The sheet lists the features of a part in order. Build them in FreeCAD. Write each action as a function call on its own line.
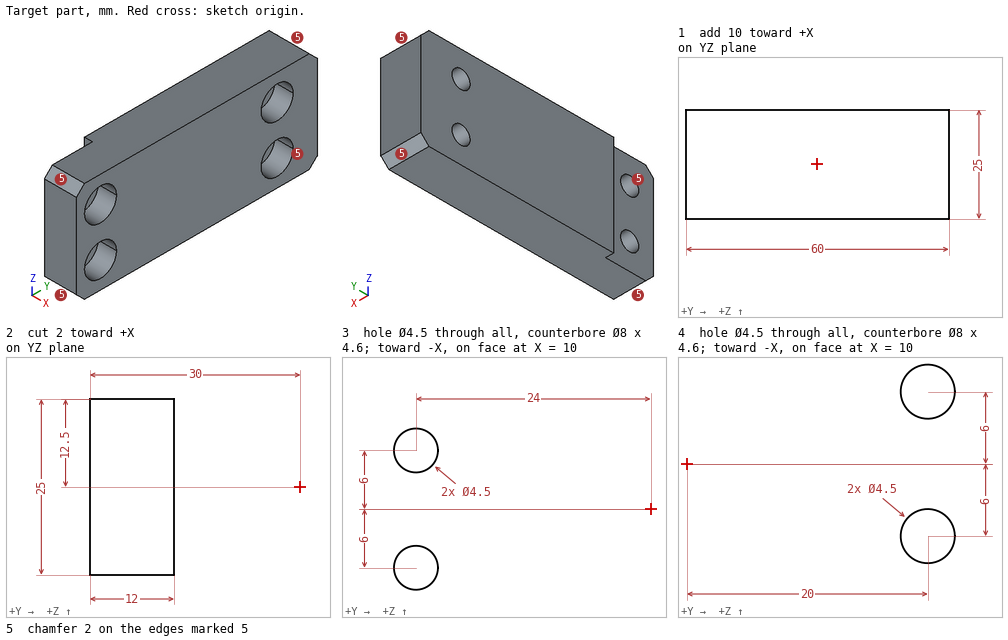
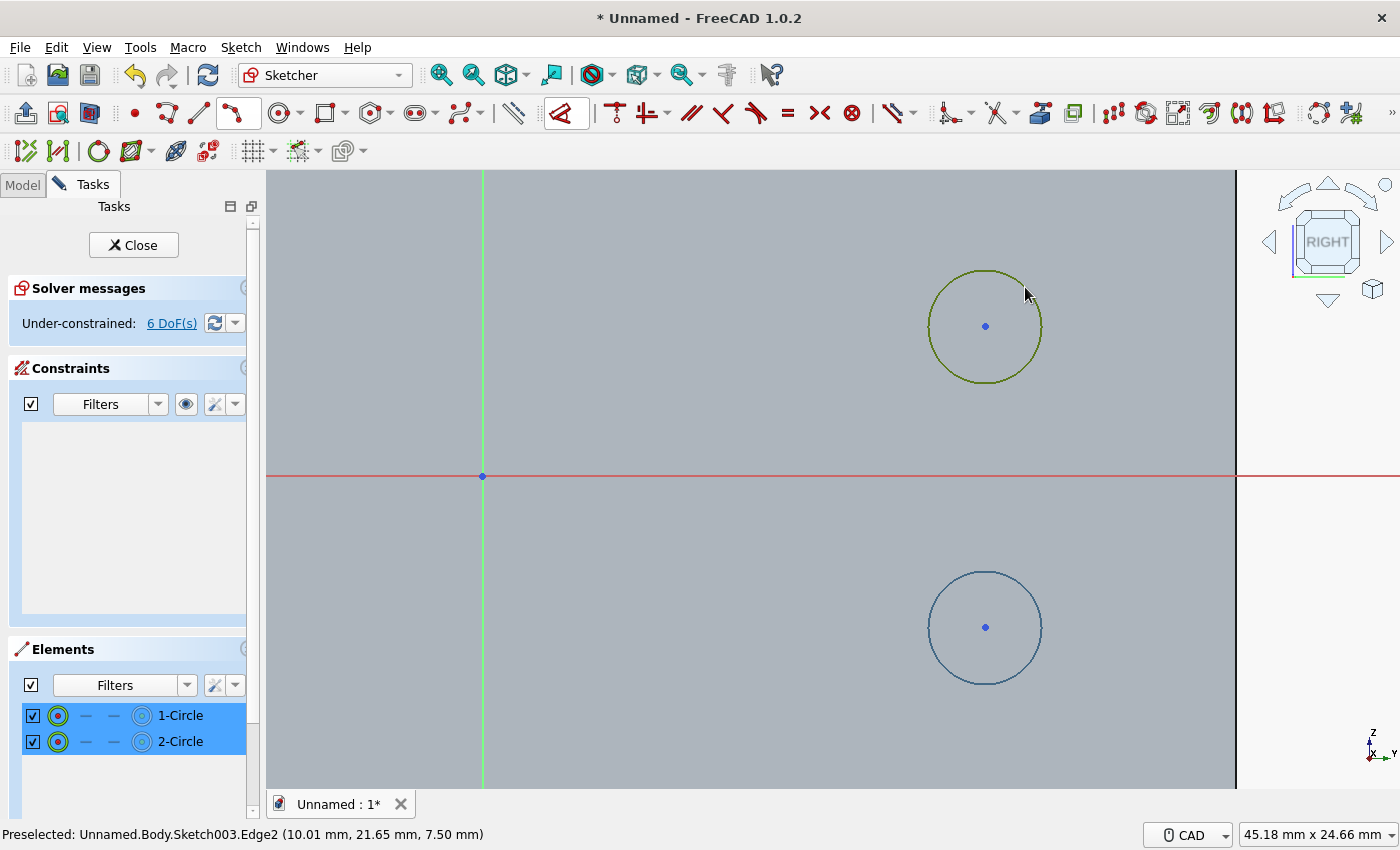
key(e)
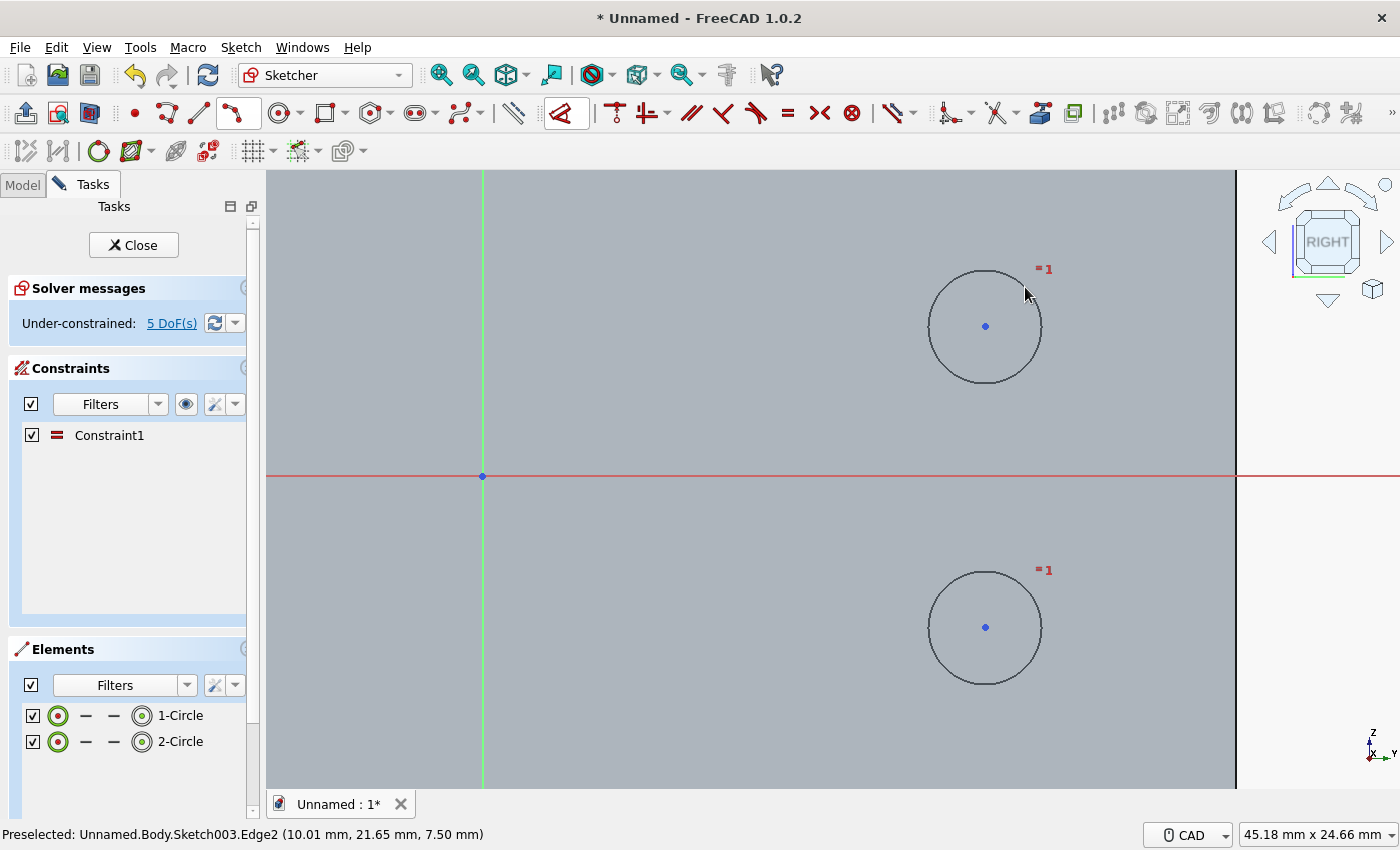
click(985, 628)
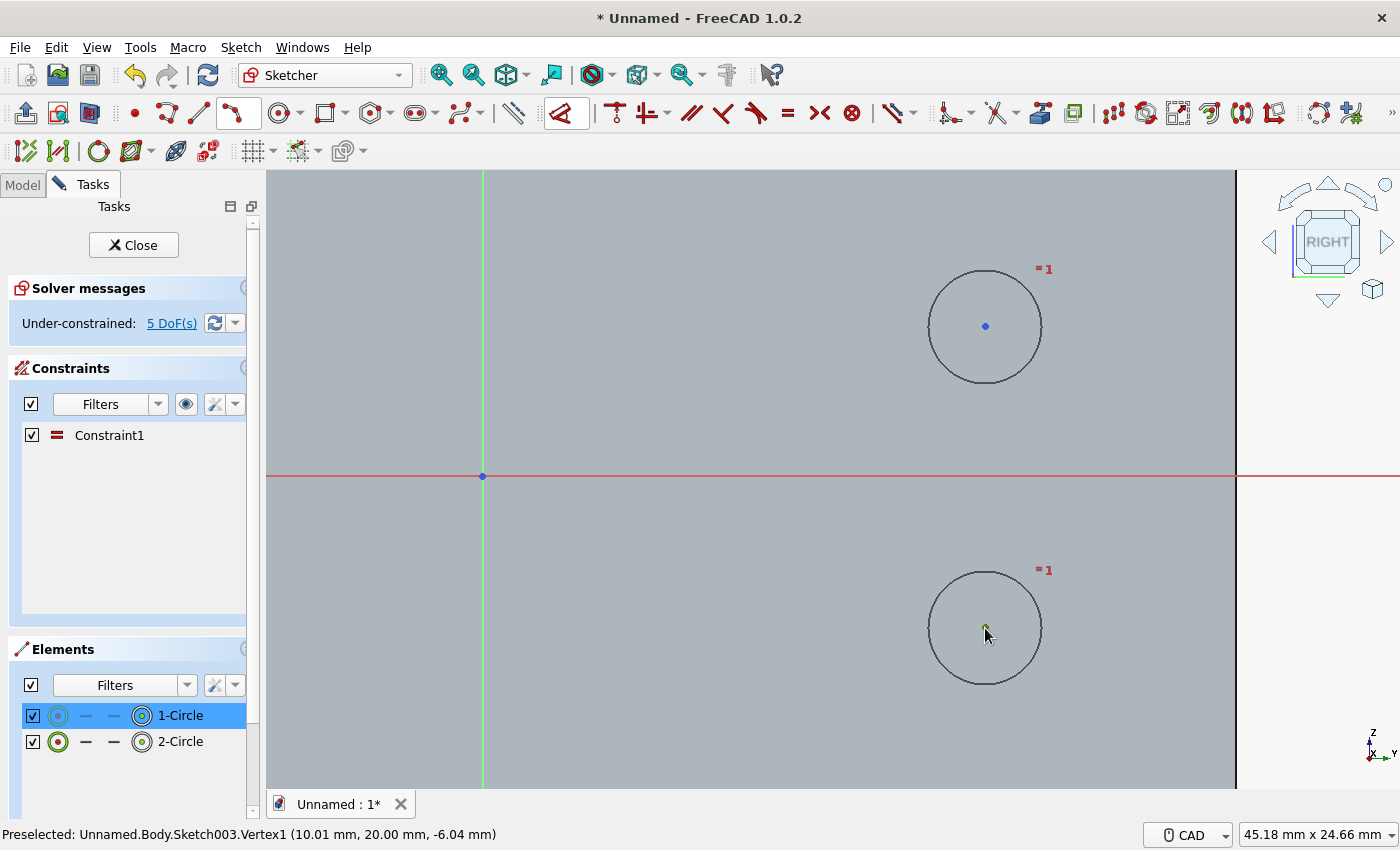
click(985, 327)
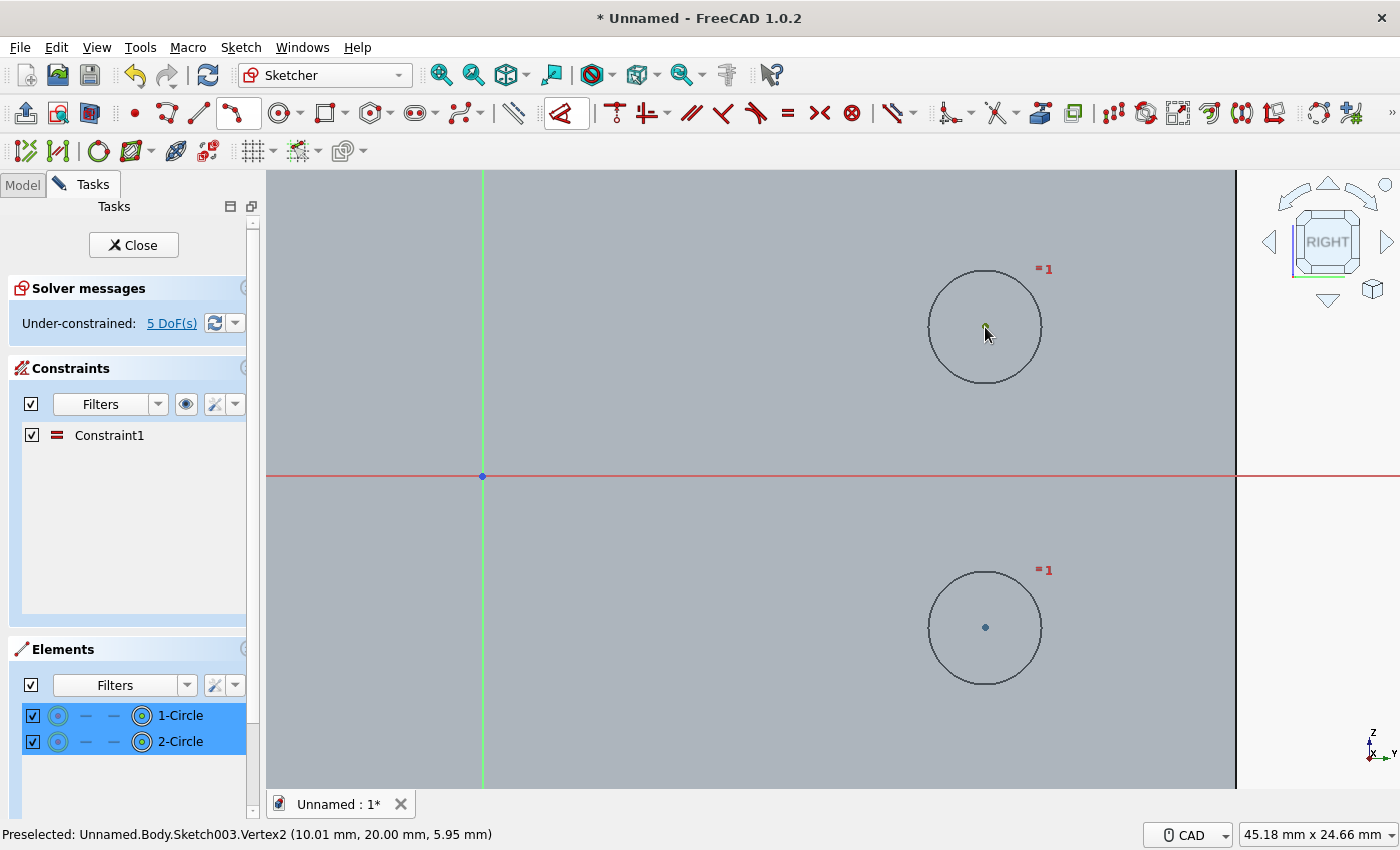
click(670, 114)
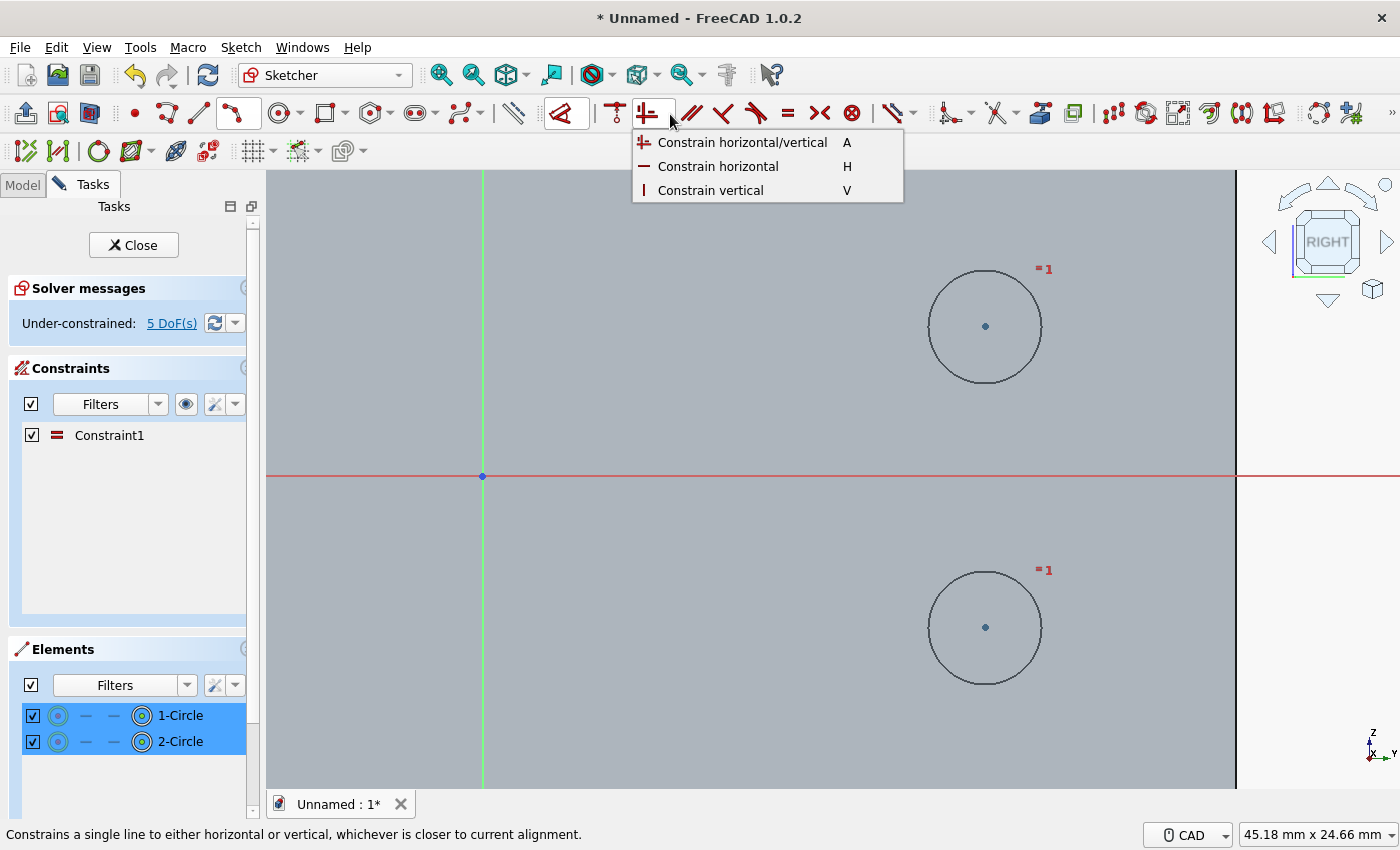
click(768, 190)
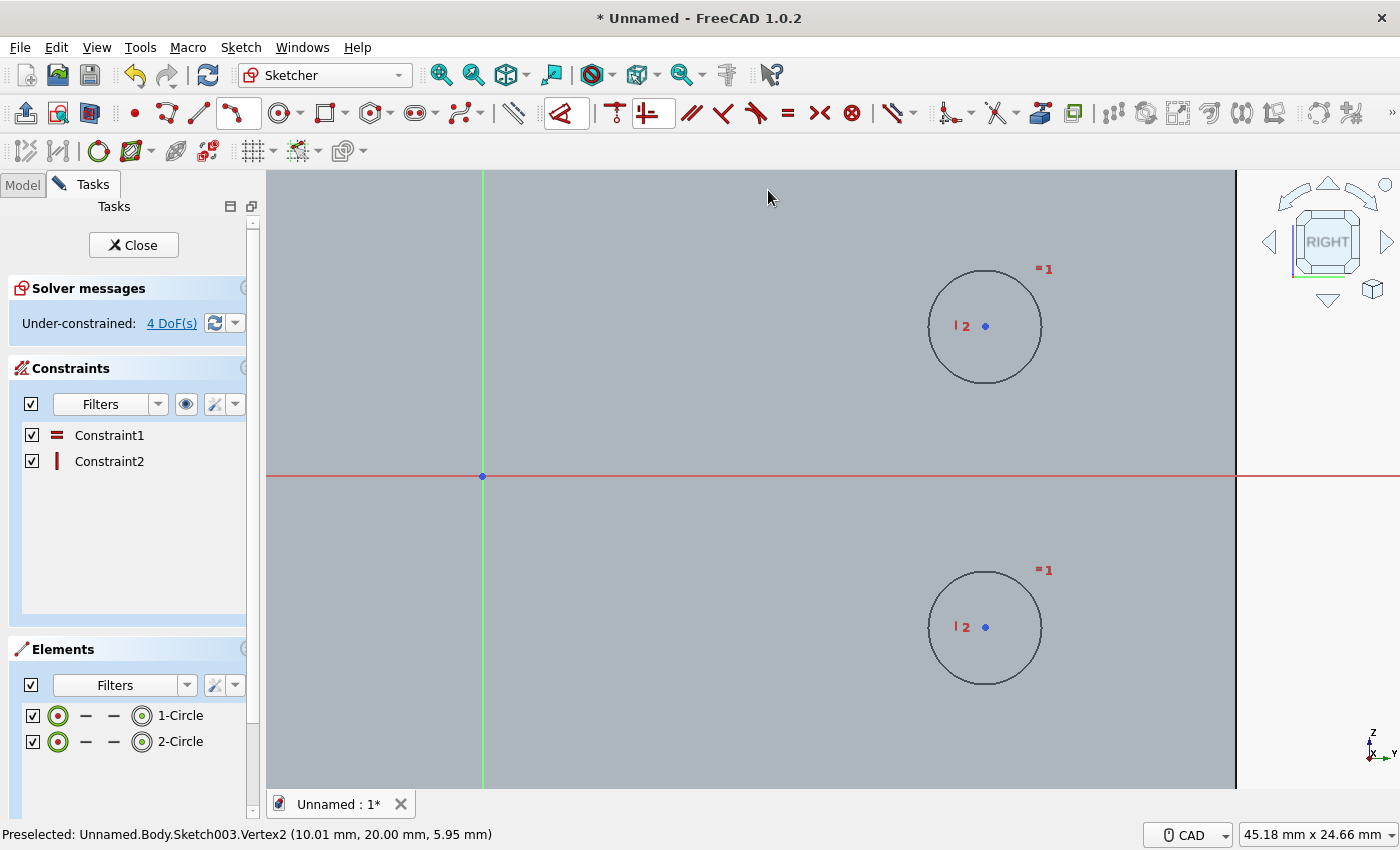
click(1025, 588)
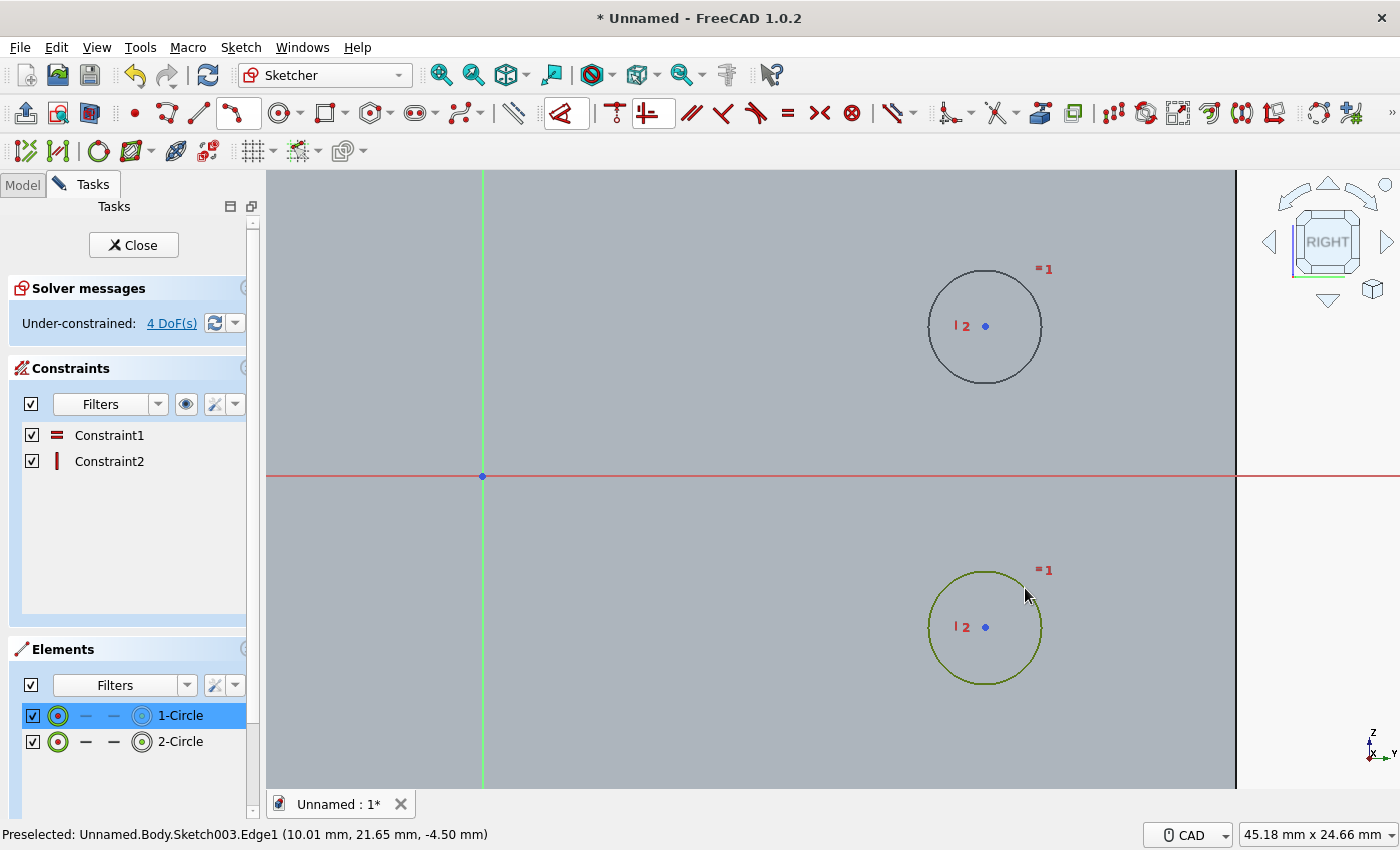
click(584, 114)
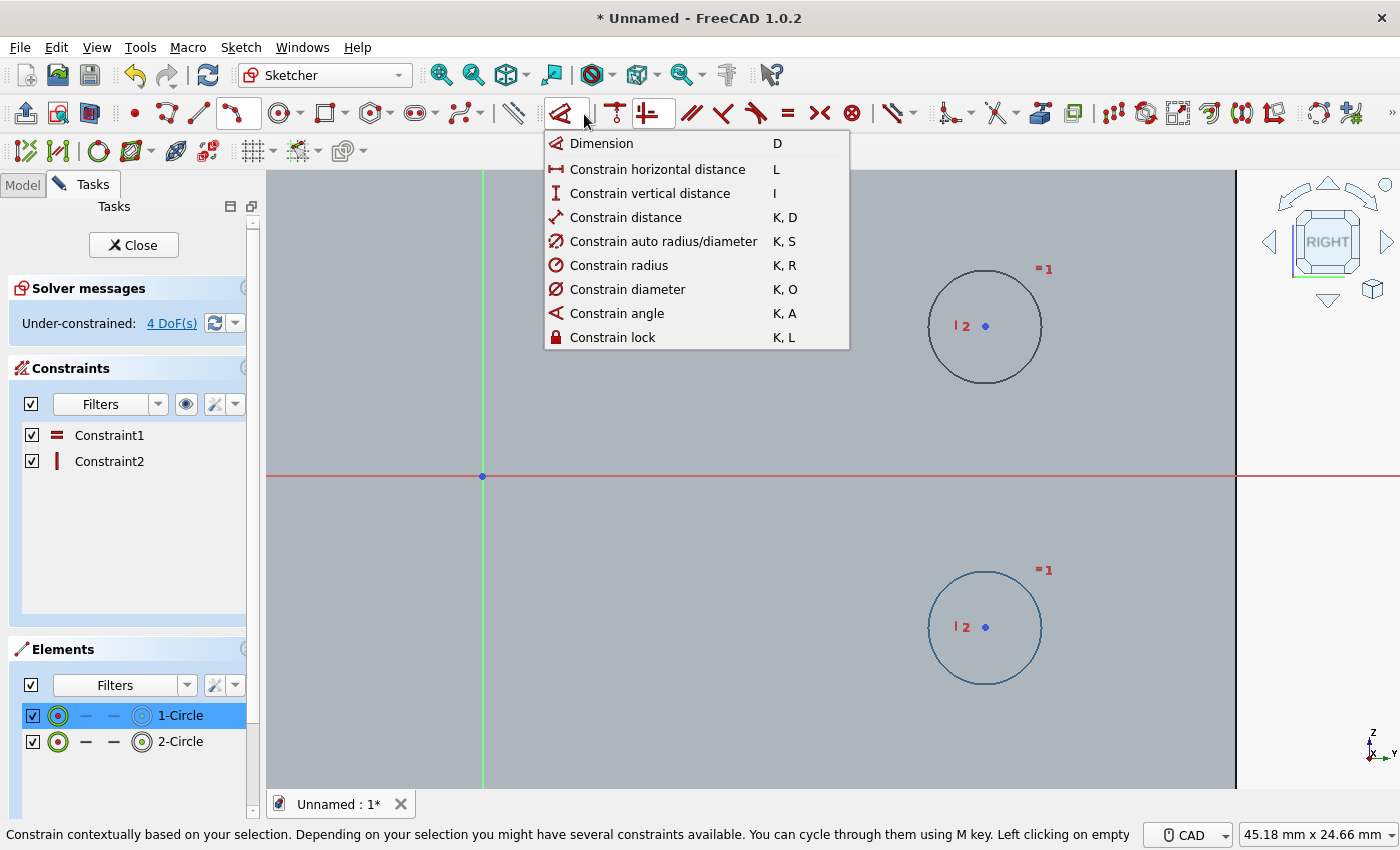
click(697, 289)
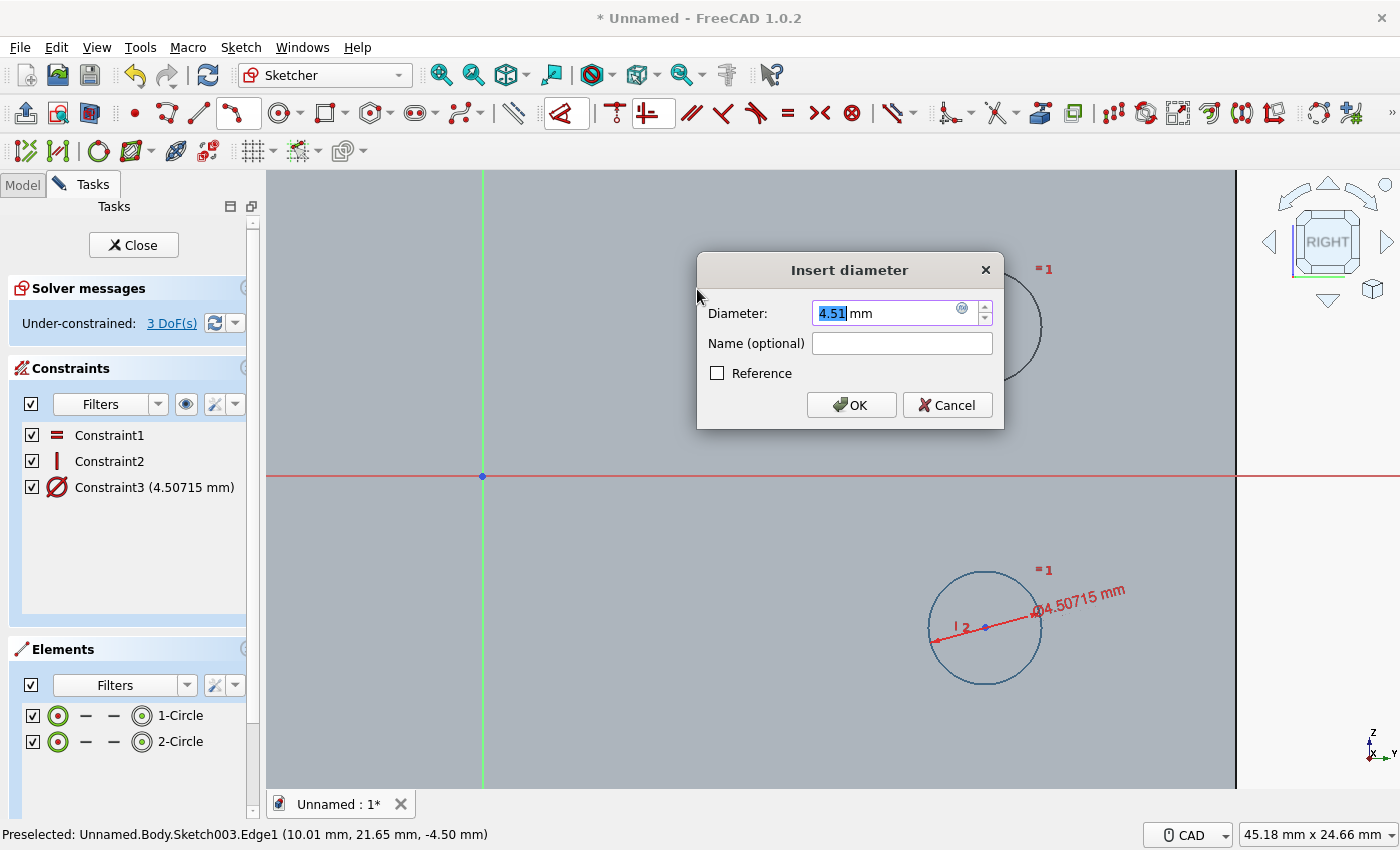
text(4.5)
key(Return)